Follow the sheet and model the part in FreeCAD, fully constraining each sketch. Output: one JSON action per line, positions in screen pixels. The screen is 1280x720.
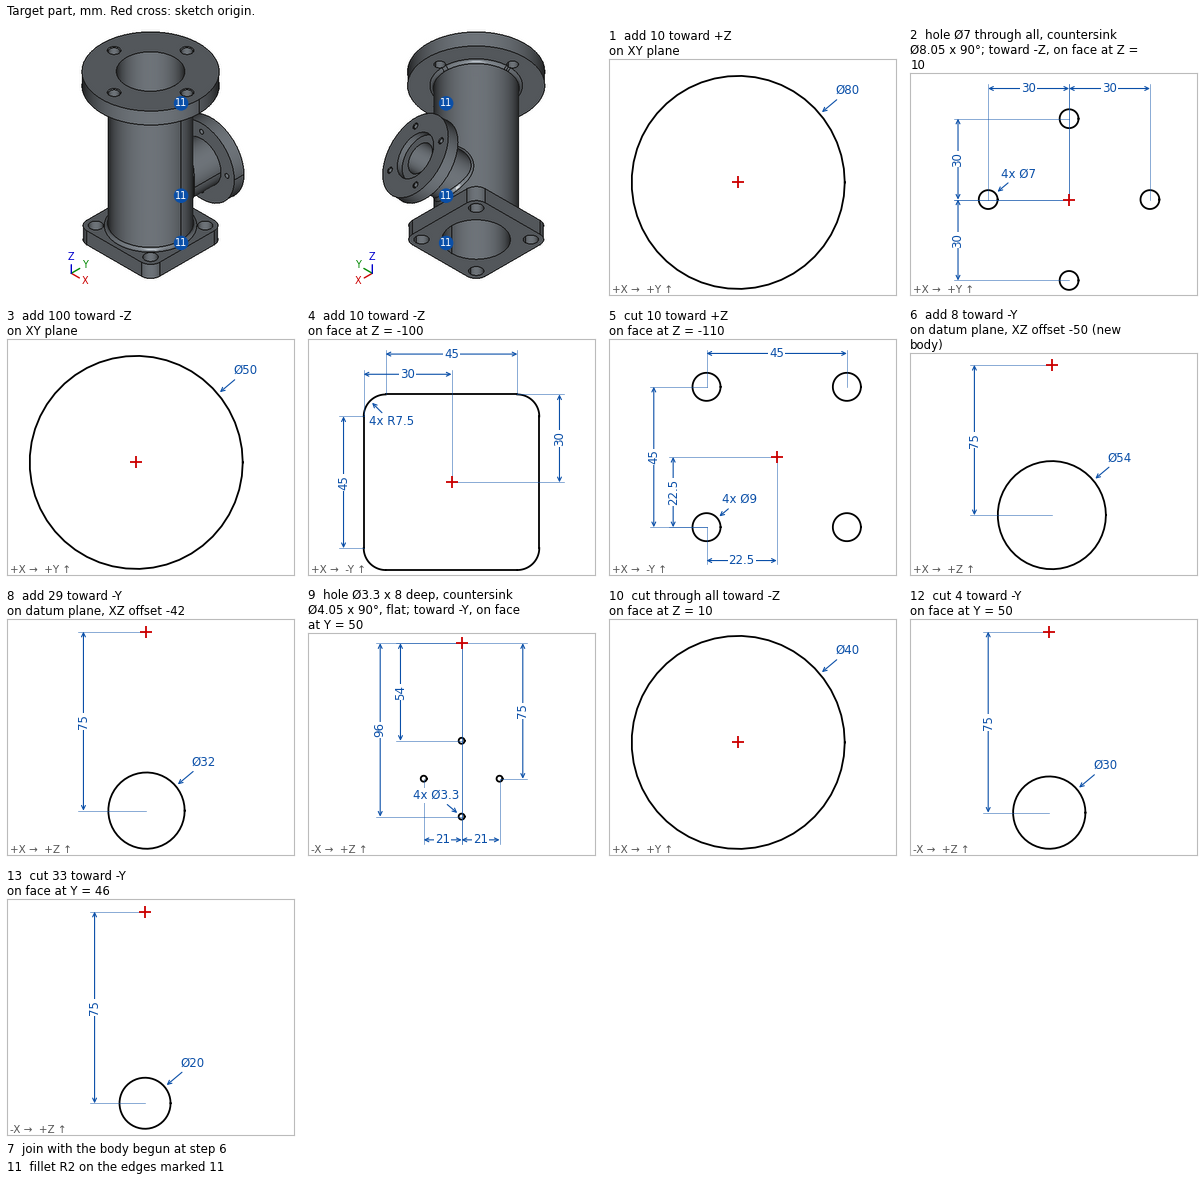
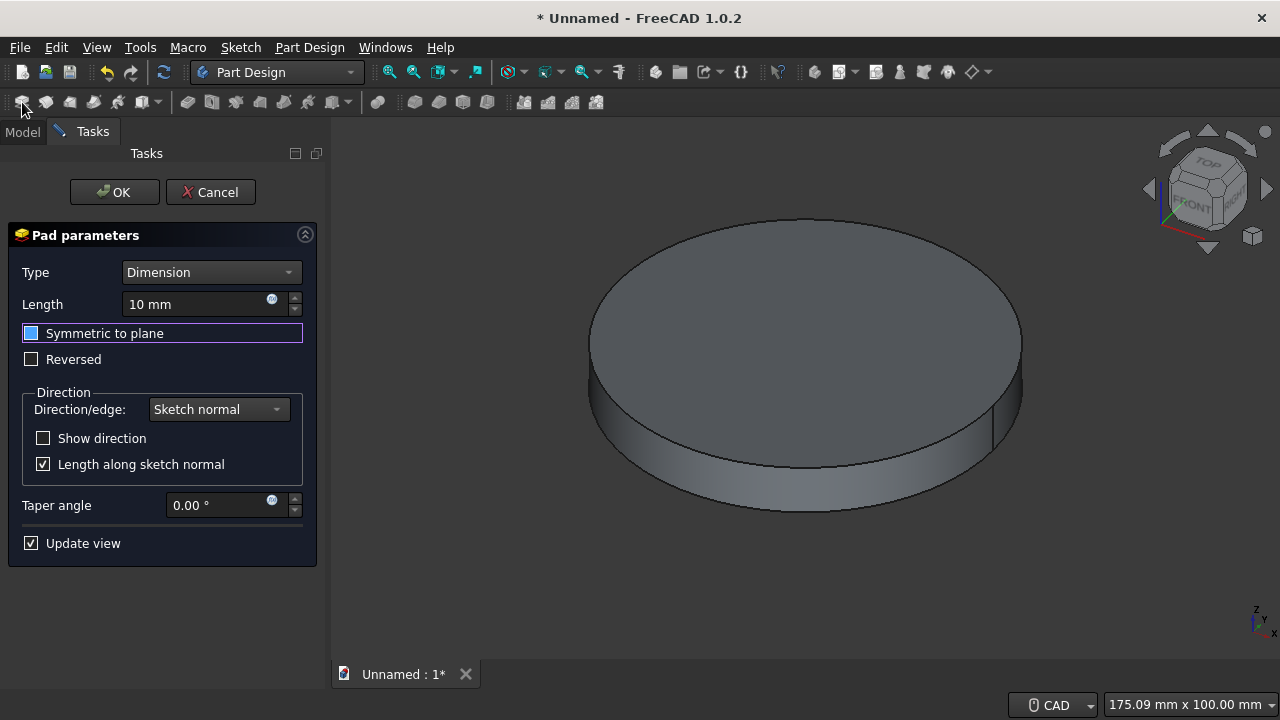
{"action": "left_click", "coordinate": [115, 192]}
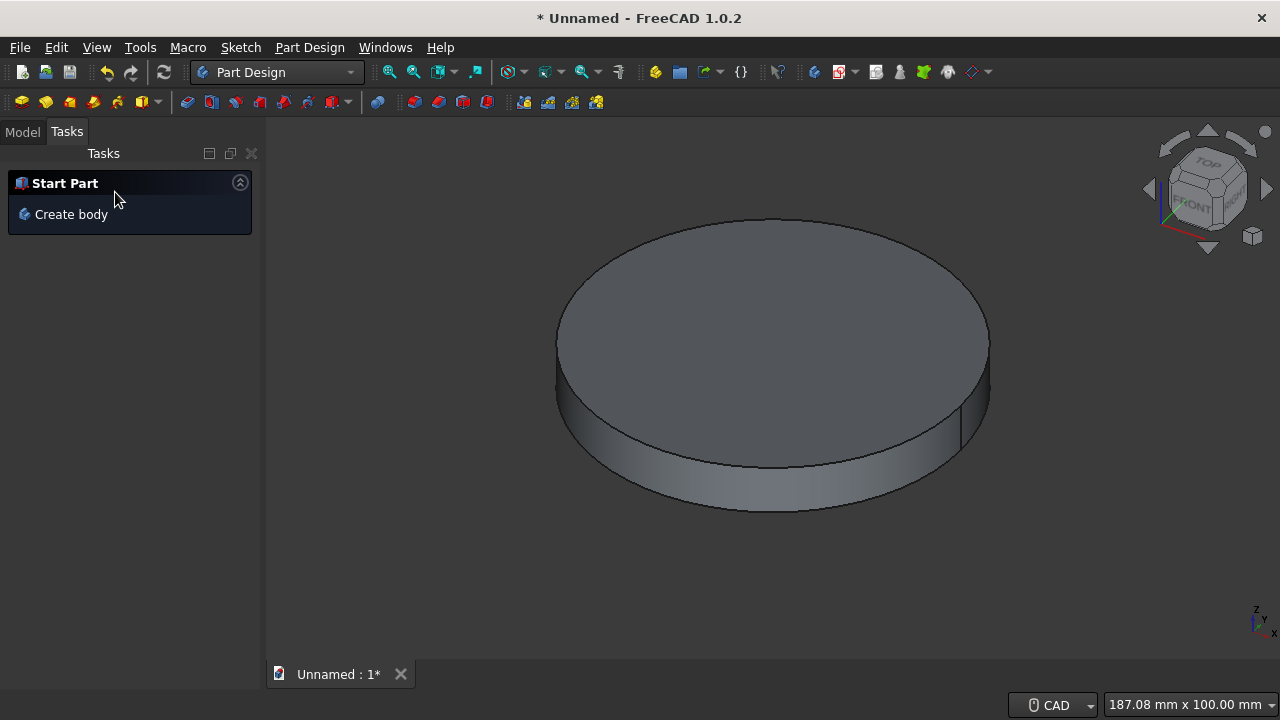
{"action": "left_click", "coordinate": [773, 343]}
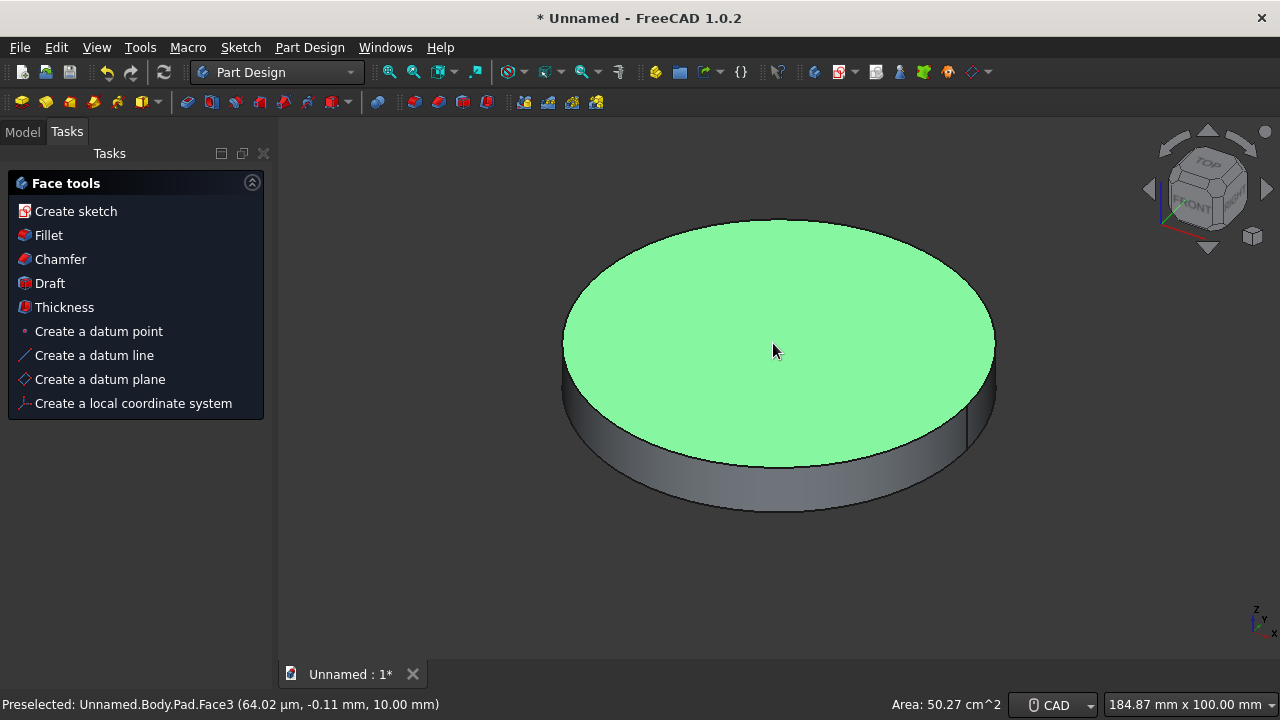
{"action": "left_click", "coordinate": [840, 72]}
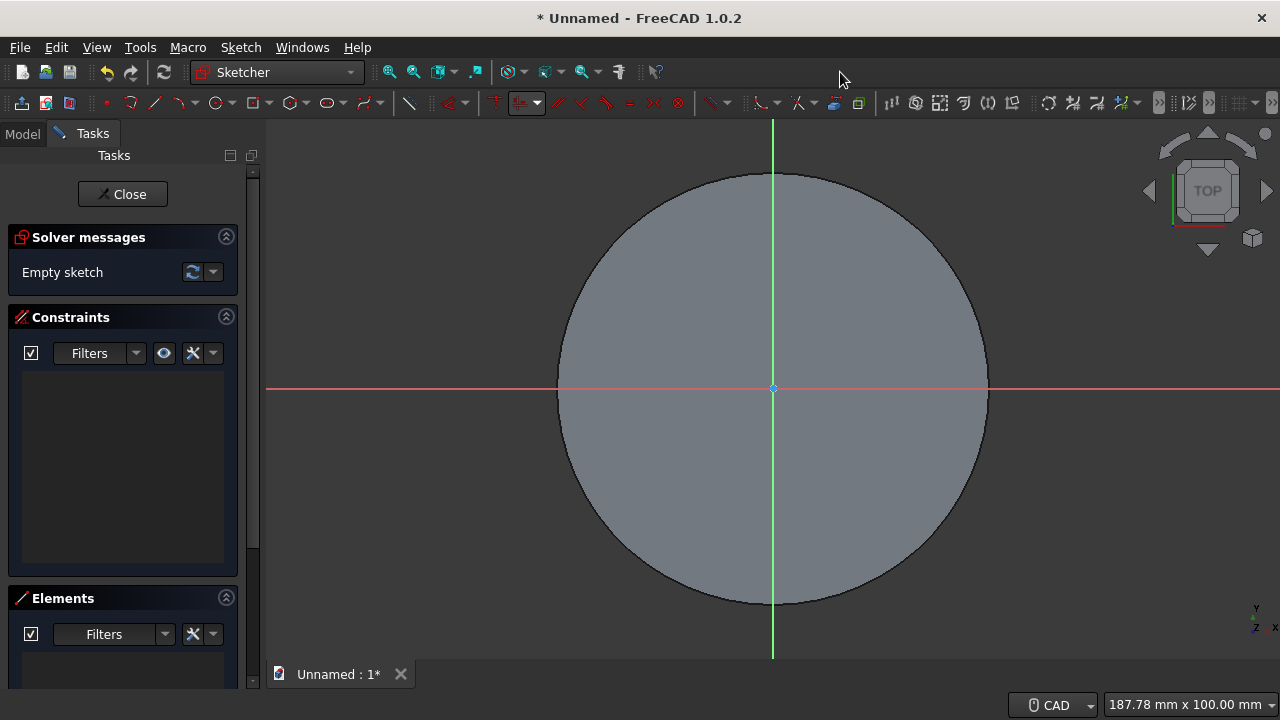
{"action": "left_click", "coordinate": [216, 104]}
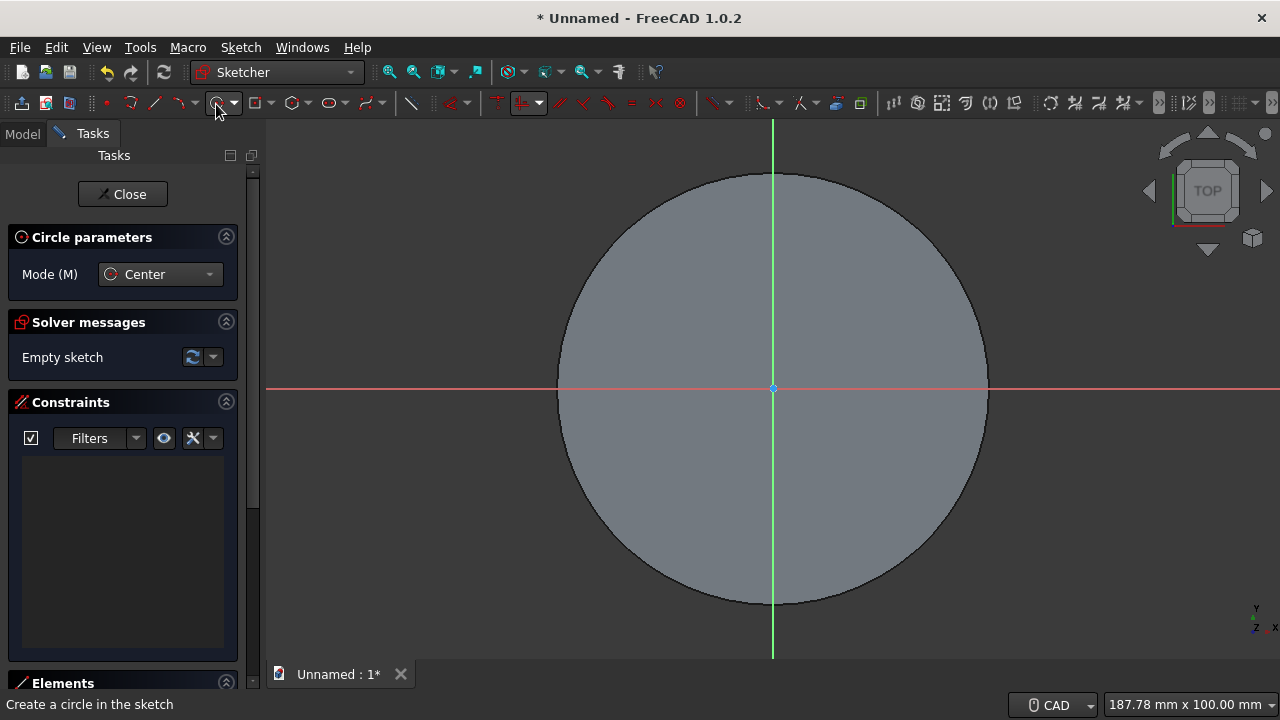
{"action": "left_click", "coordinate": [611, 389]}
{"action": "mouse_move", "coordinate": [617, 371]}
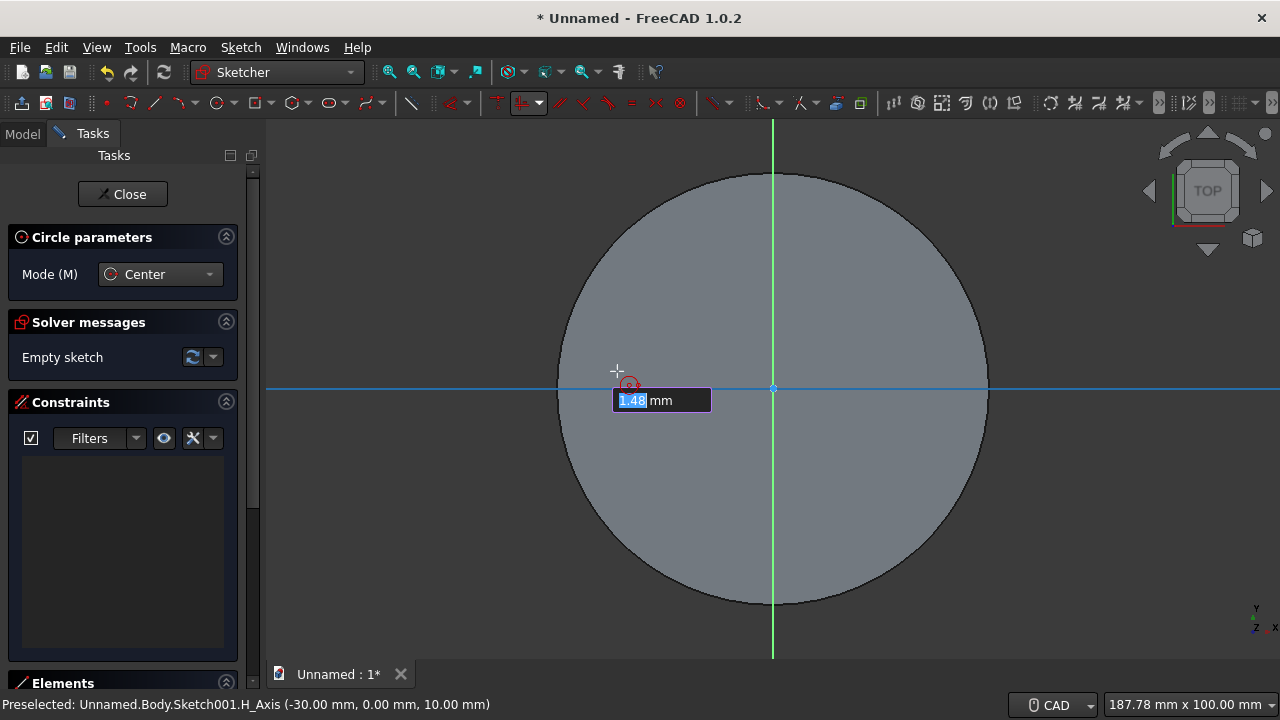
{"action": "type", "text": "7"}
{"action": "key", "text": "Return"}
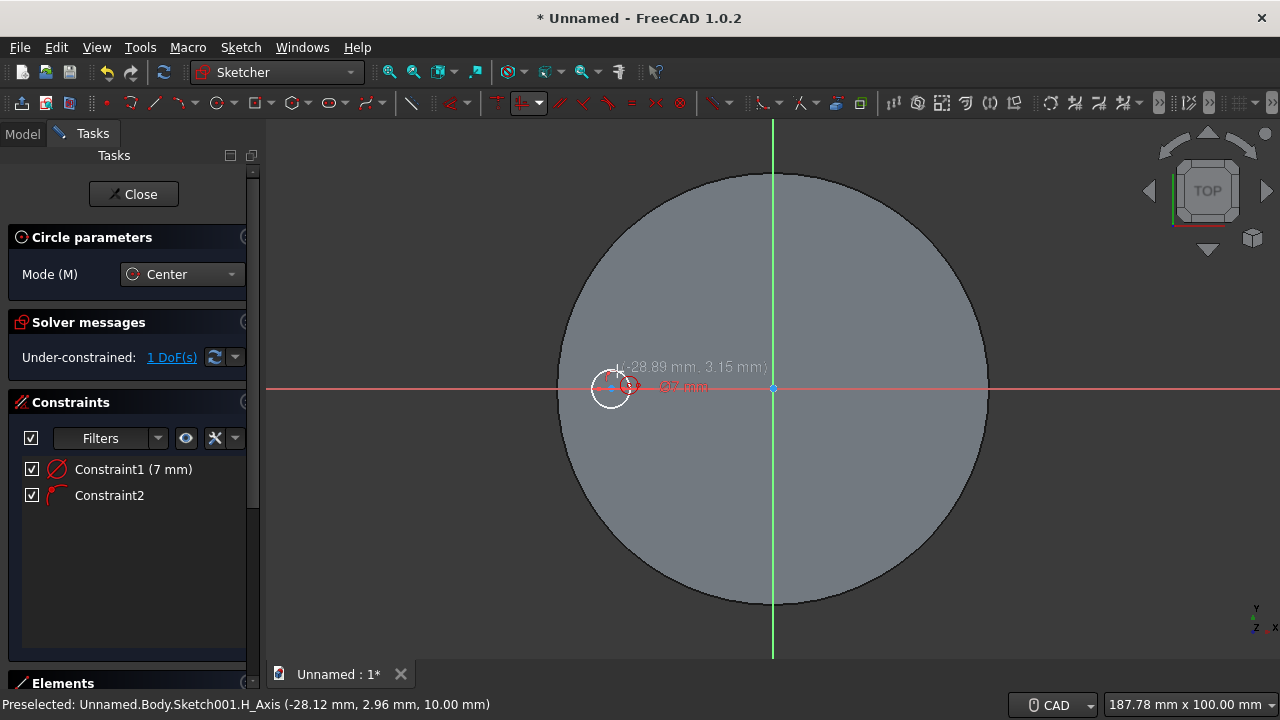
{"action": "left_click", "coordinate": [935, 389]}
{"action": "mouse_move", "coordinate": [941, 371]}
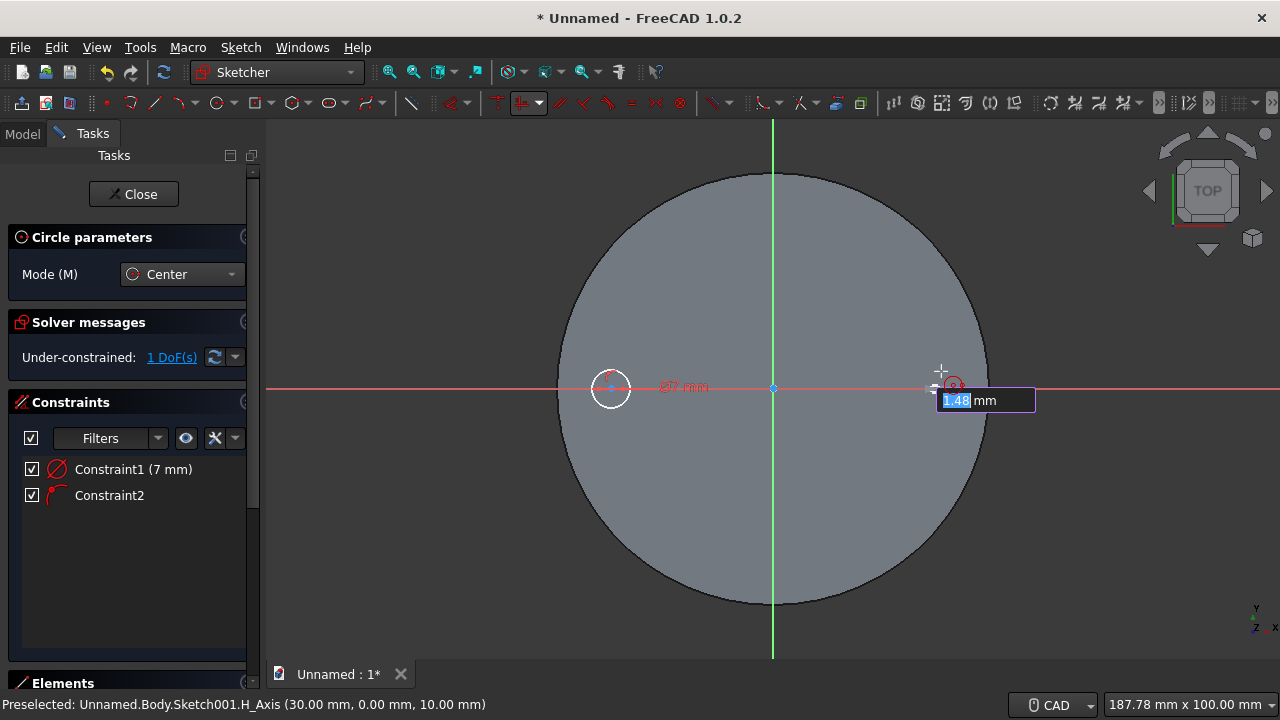
{"action": "type", "text": "7"}
{"action": "key", "text": "Return"}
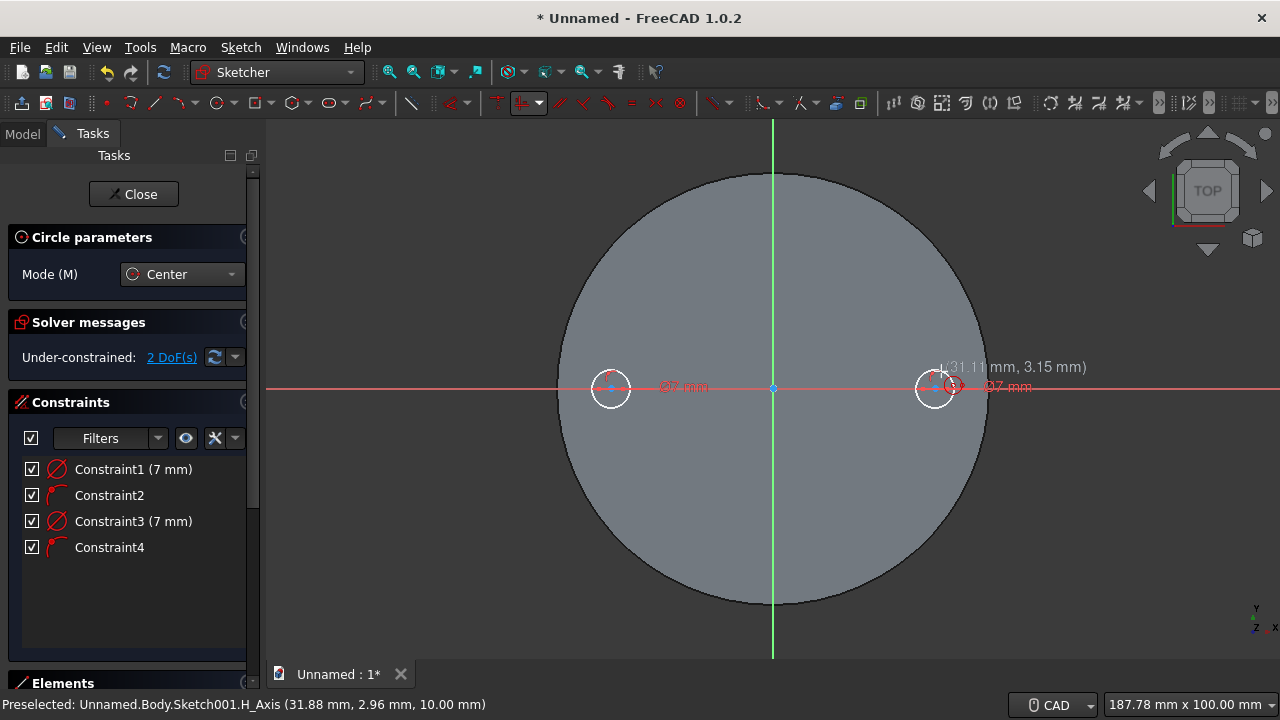
{"action": "left_click", "coordinate": [773, 227]}
{"action": "mouse_move", "coordinate": [791, 221]}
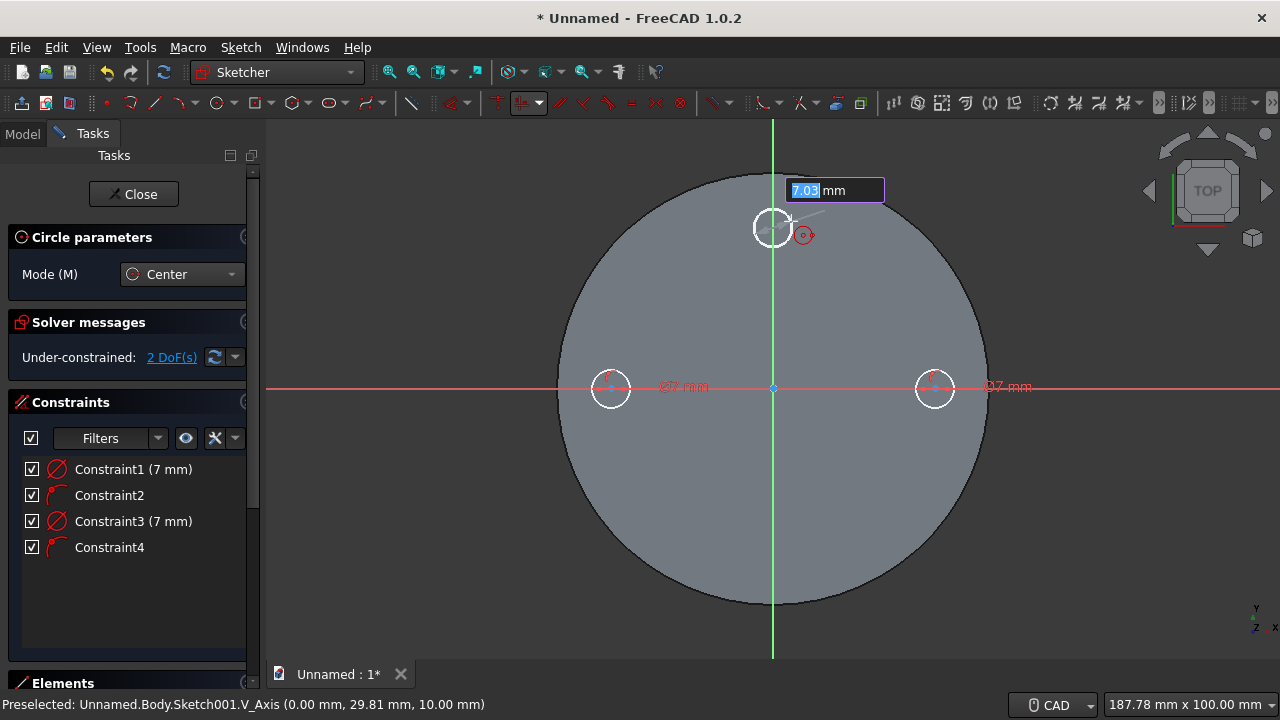
{"action": "type", "text": "7"}
{"action": "key", "text": "Return"}